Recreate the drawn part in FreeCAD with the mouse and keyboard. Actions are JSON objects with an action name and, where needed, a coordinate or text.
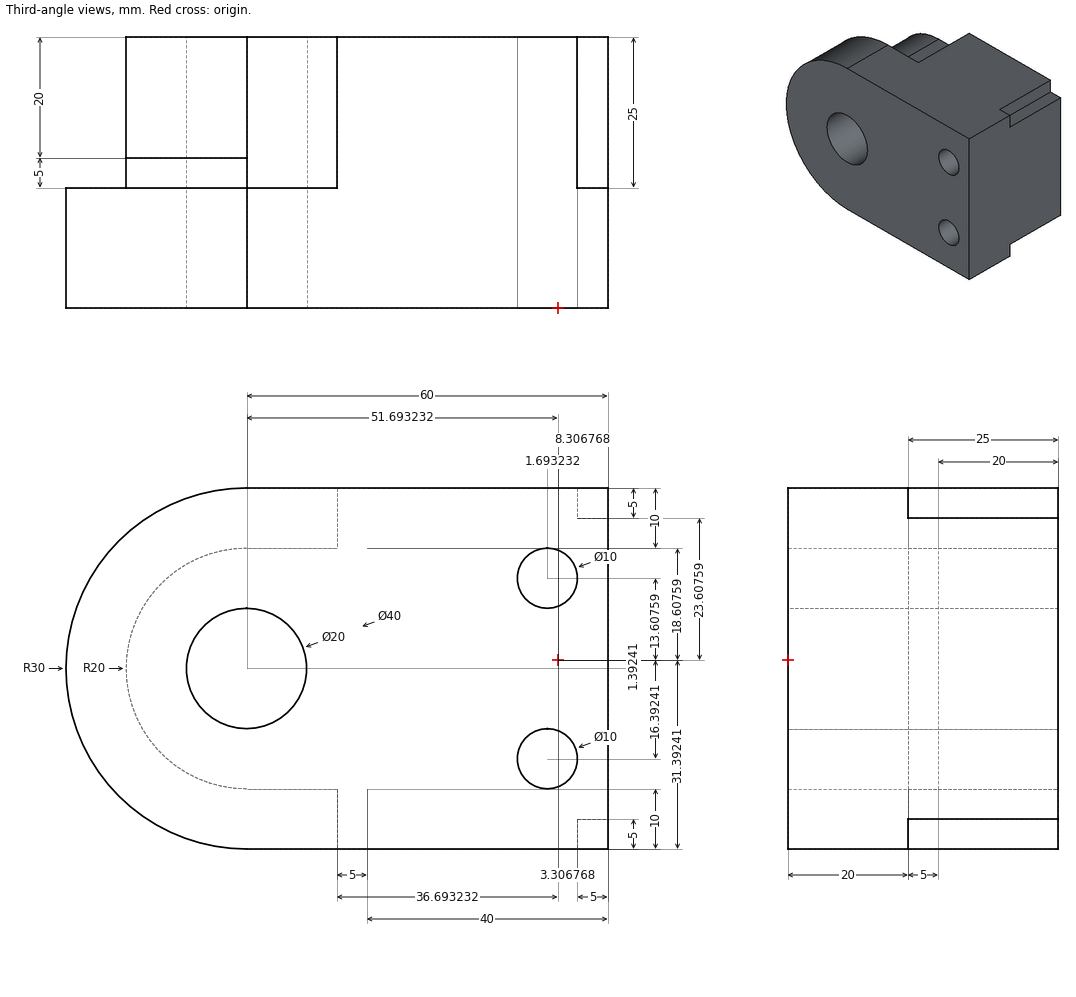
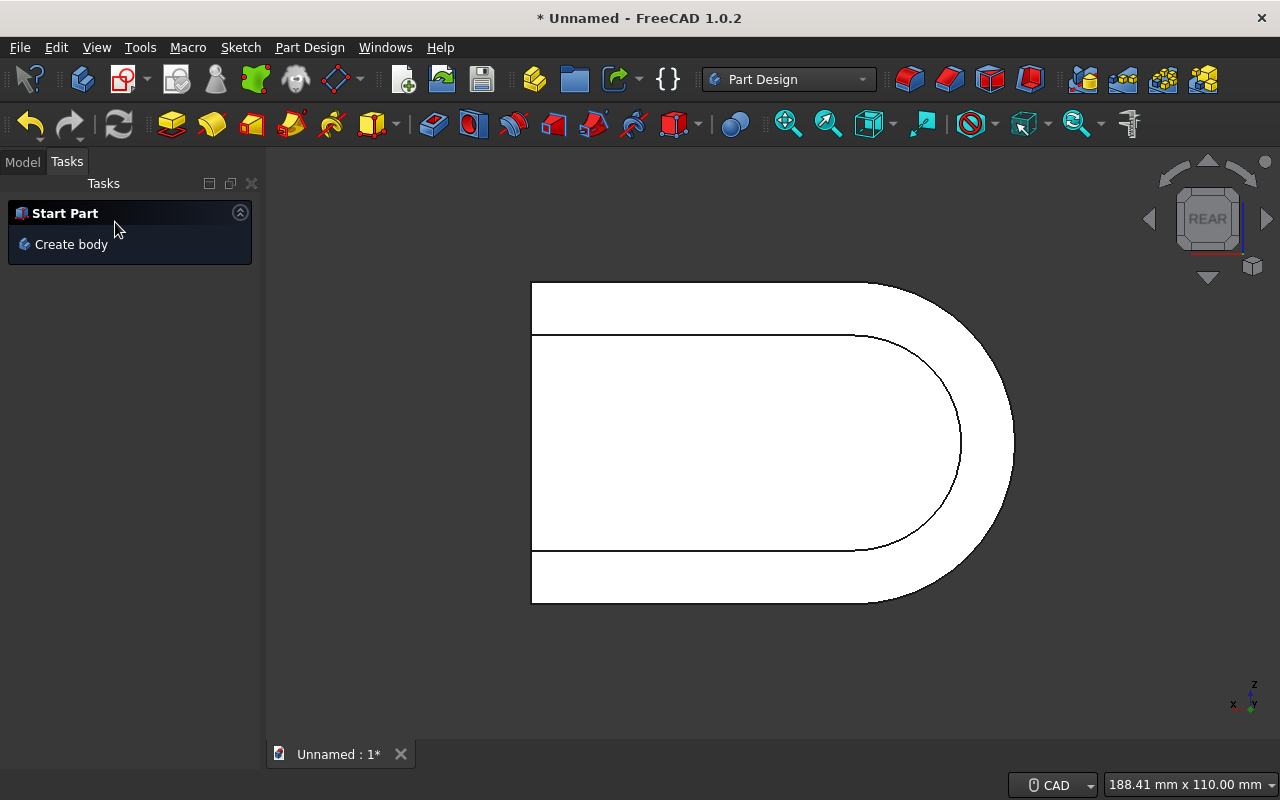
{"action": "left_click", "coordinate": [981, 396]}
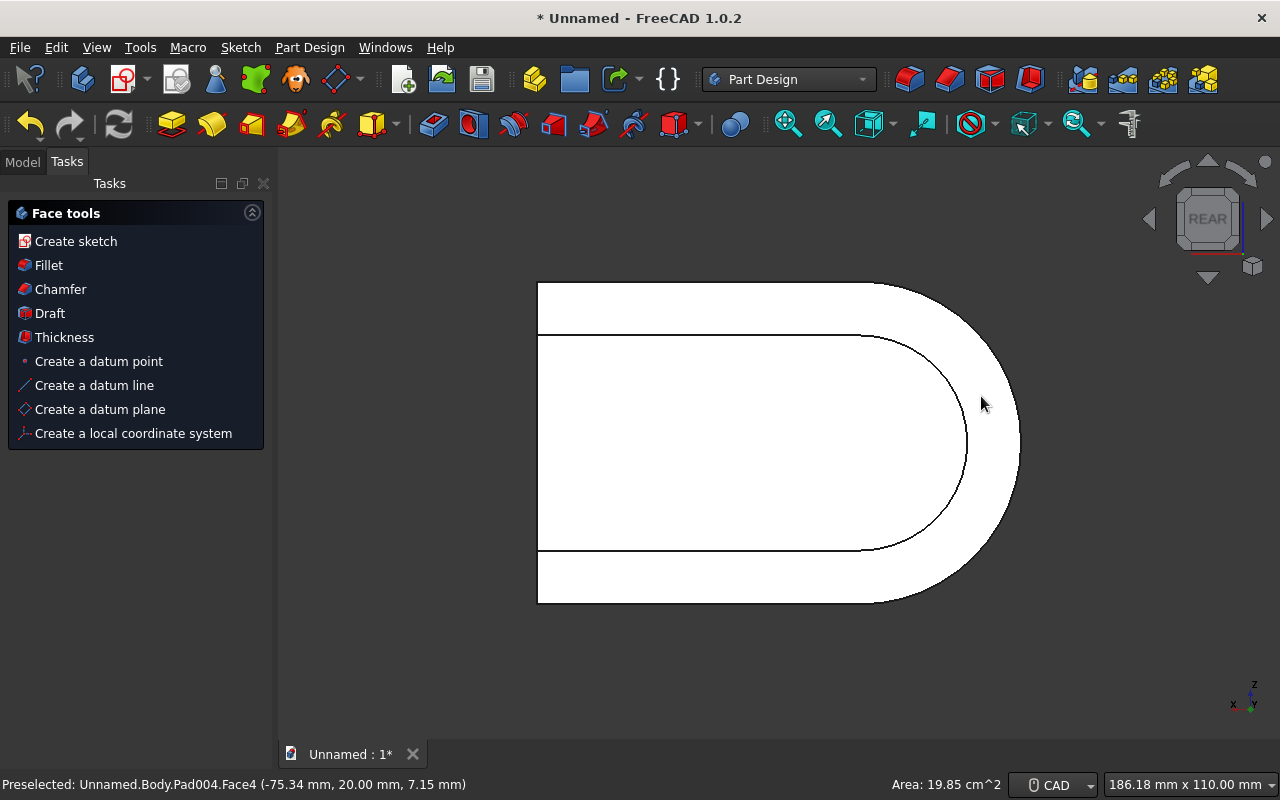
{"action": "left_click", "coordinate": [124, 80]}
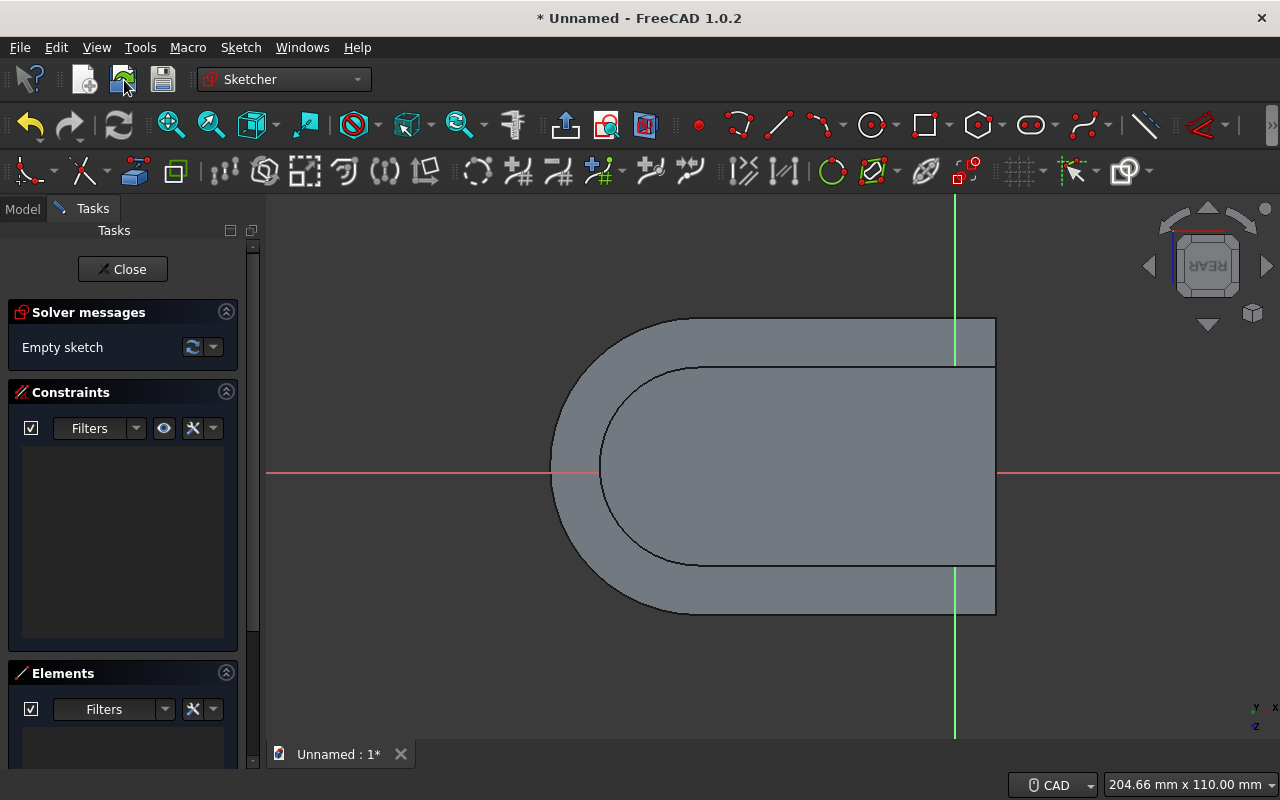
{"action": "key", "text": "q s"}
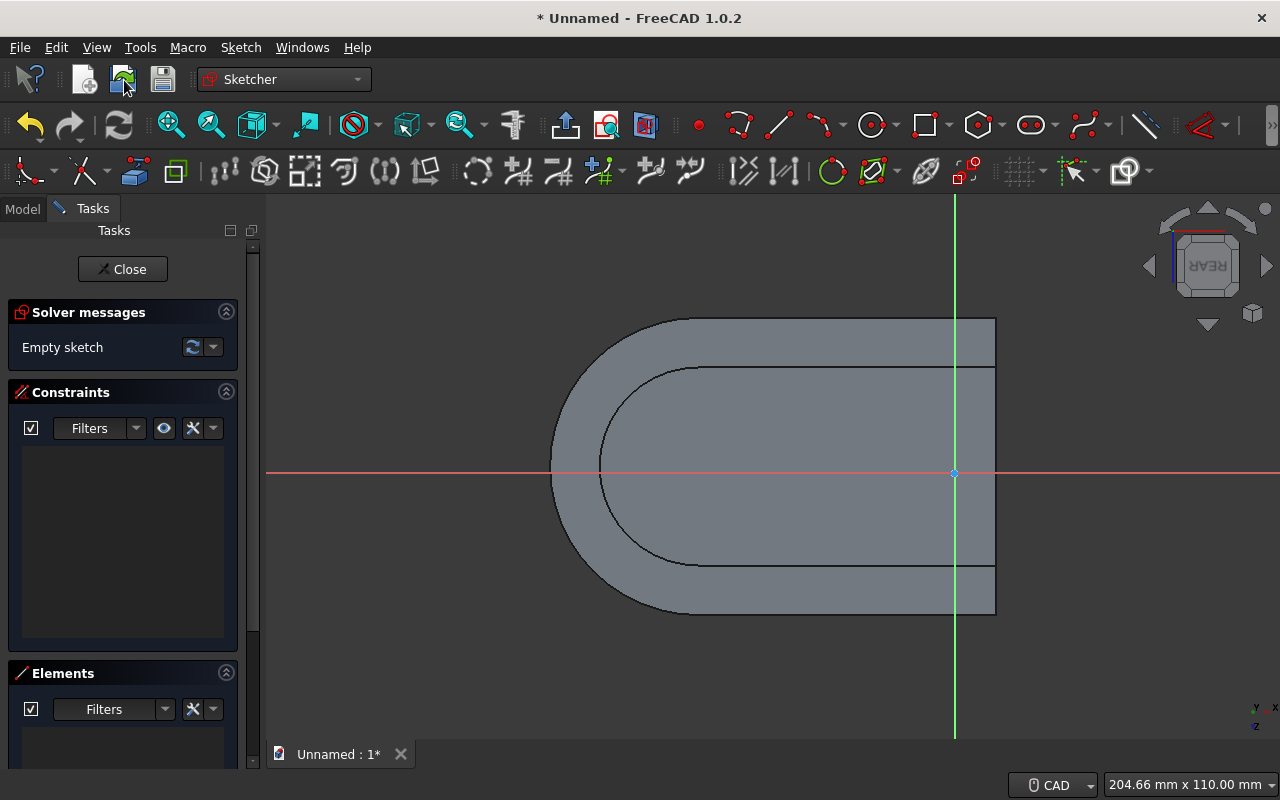
{"action": "scroll", "coordinate": [1054, 338], "scroll_direction": "up", "scroll_amount": 4}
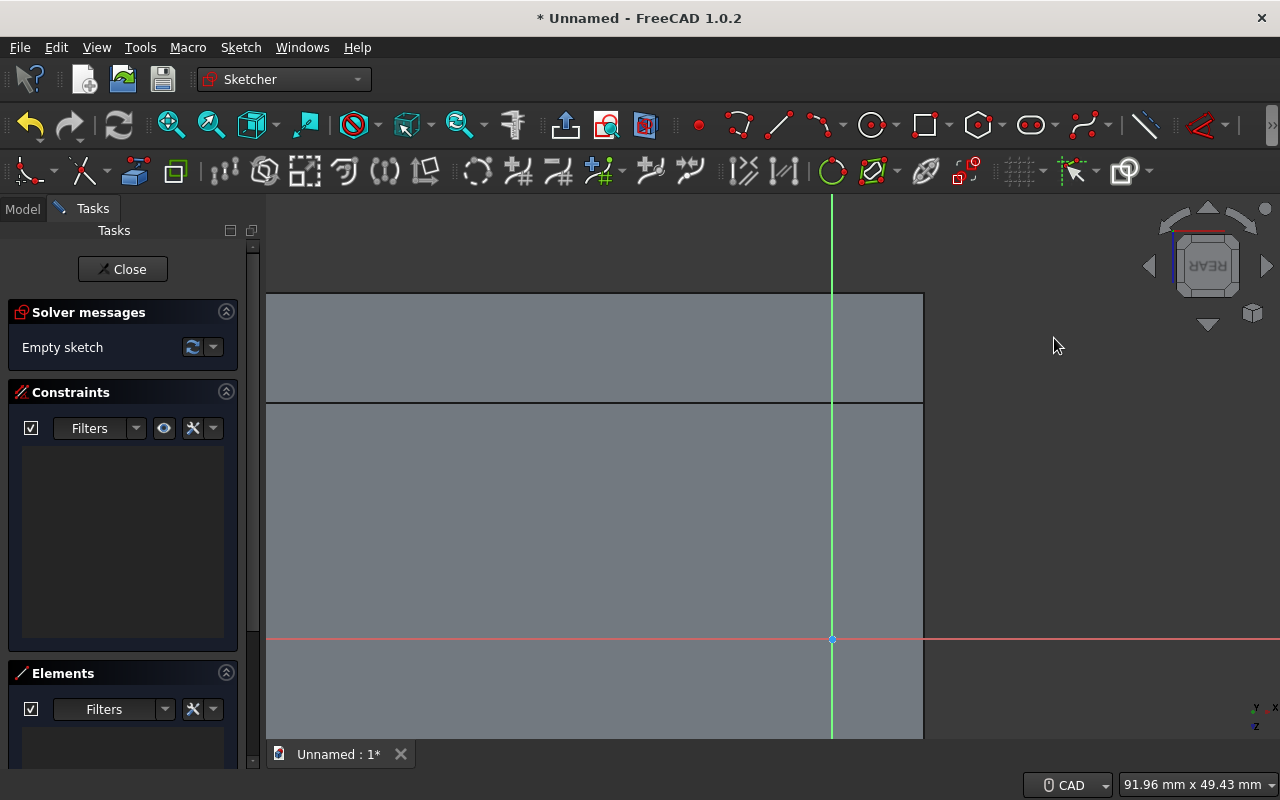
{"action": "key", "text": "g r"}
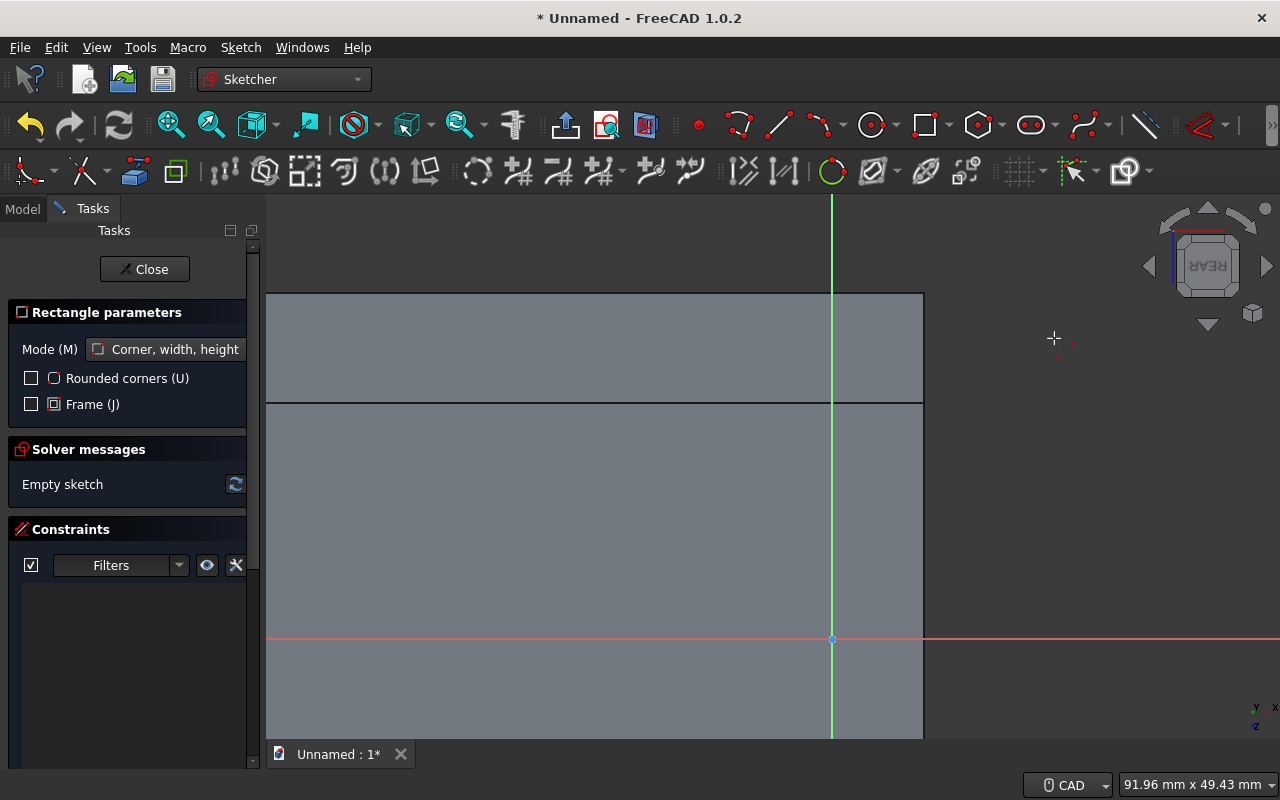
{"action": "left_click", "coordinate": [483, 293]}
{"action": "left_click", "coordinate": [924, 403]}
{"action": "key", "text": "Escape"}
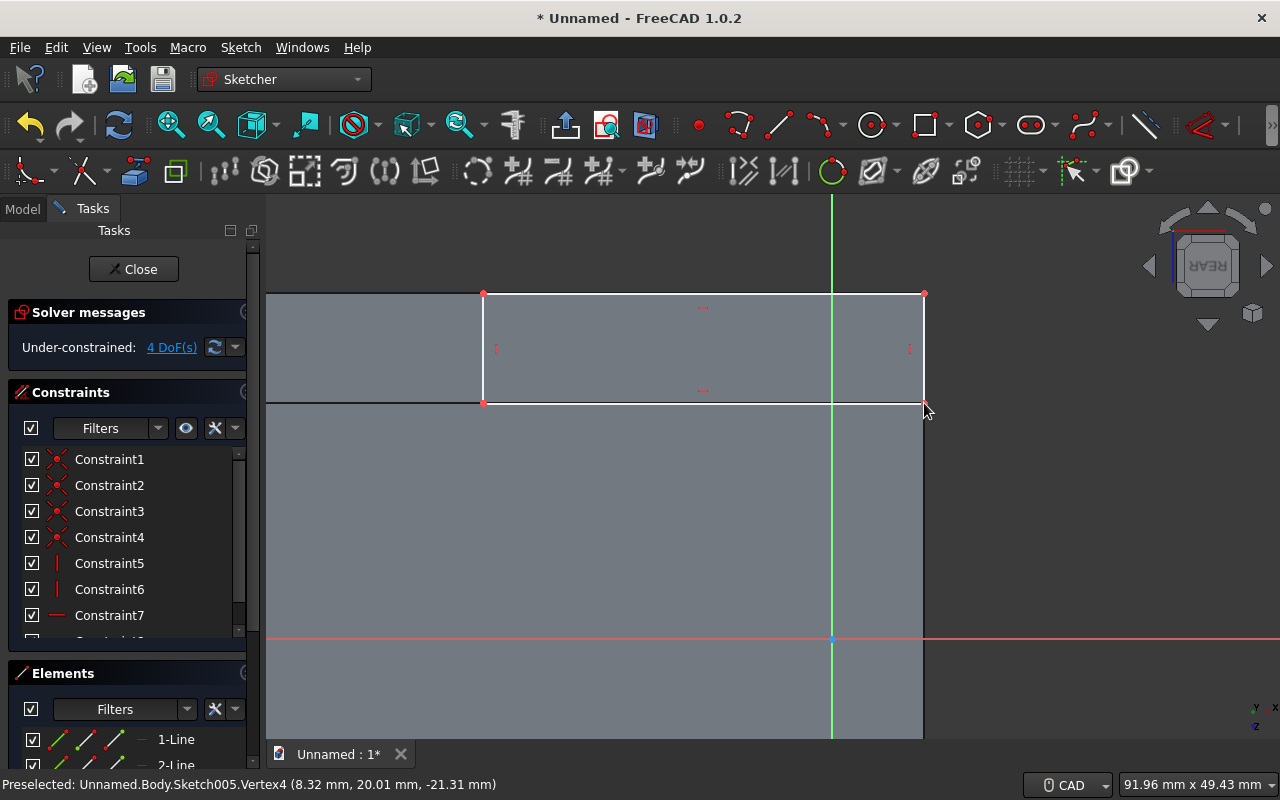
{"action": "key", "text": "d"}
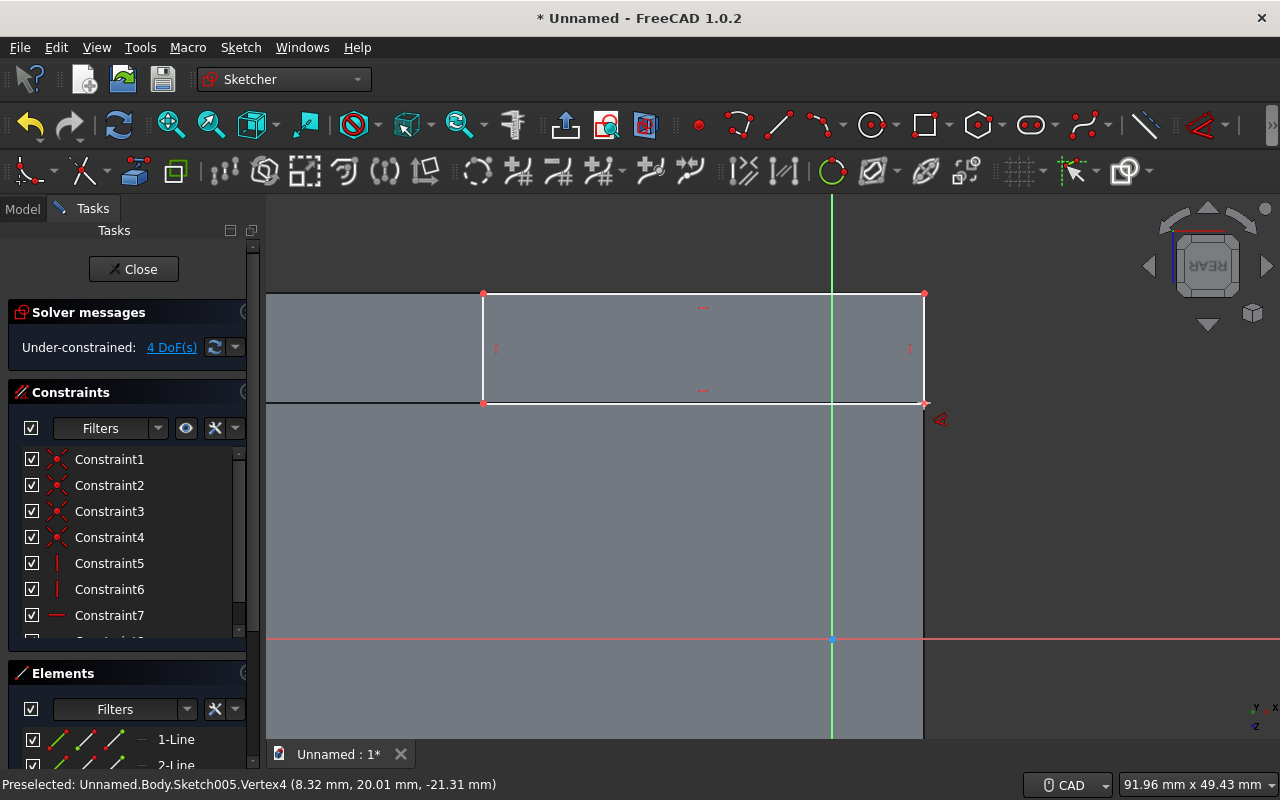
{"action": "left_click", "coordinate": [483, 327]}
{"action": "left_click", "coordinate": [449, 349]}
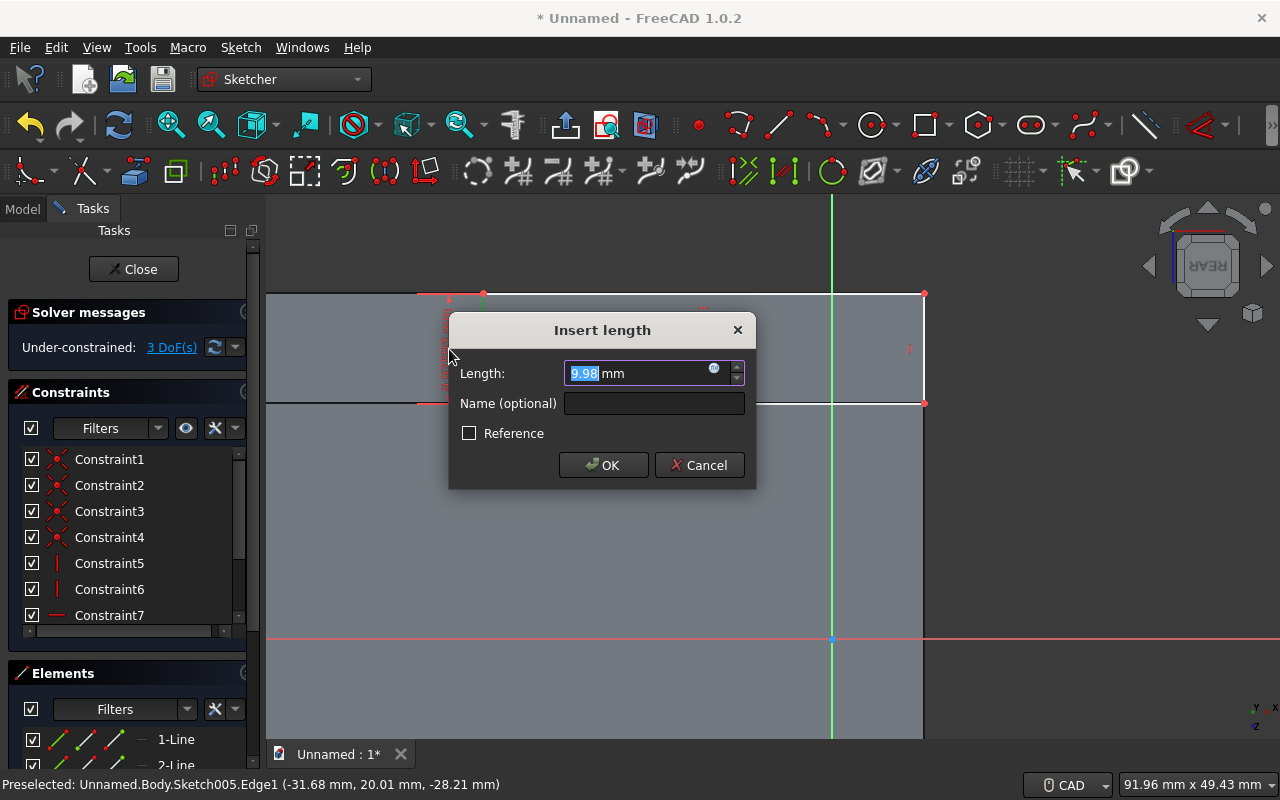
{"action": "type", "text": "10"}
{"action": "key", "text": "Return"}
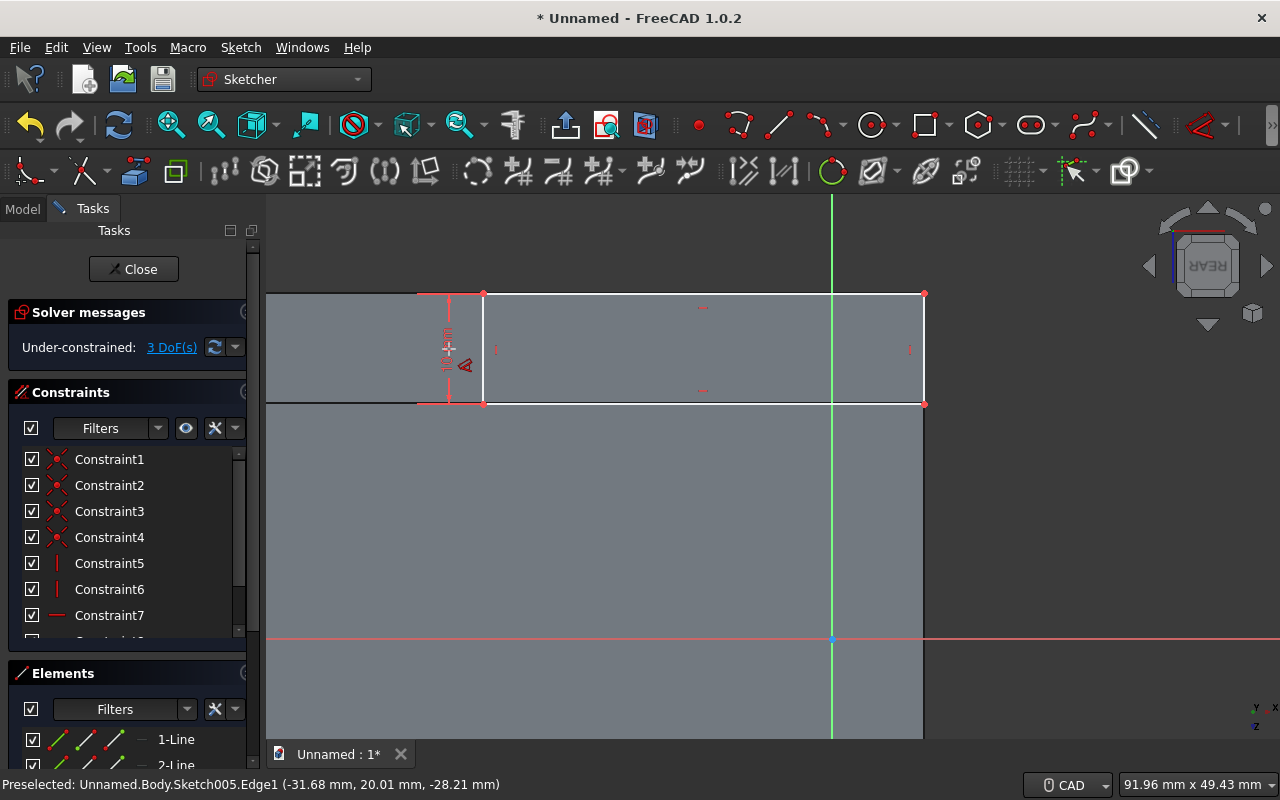
{"action": "left_click", "coordinate": [615, 404]}
{"action": "left_click", "coordinate": [703, 370]}